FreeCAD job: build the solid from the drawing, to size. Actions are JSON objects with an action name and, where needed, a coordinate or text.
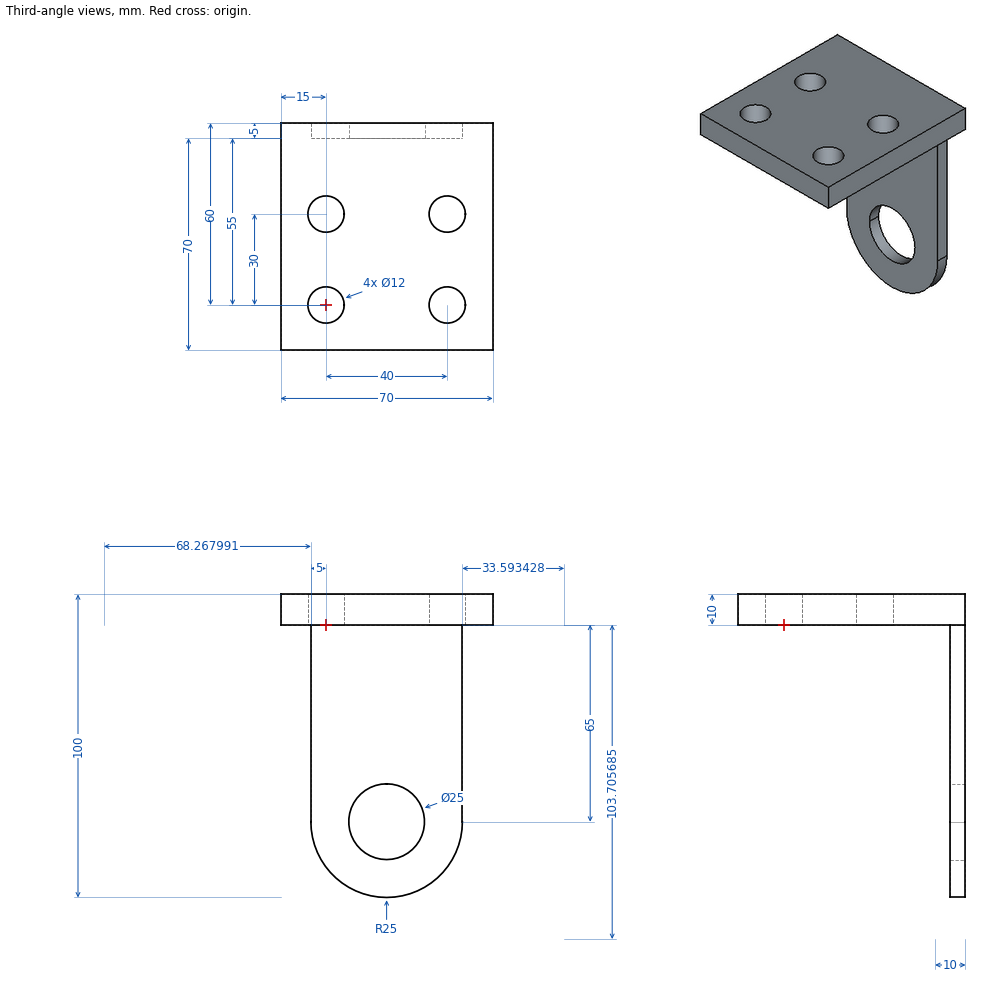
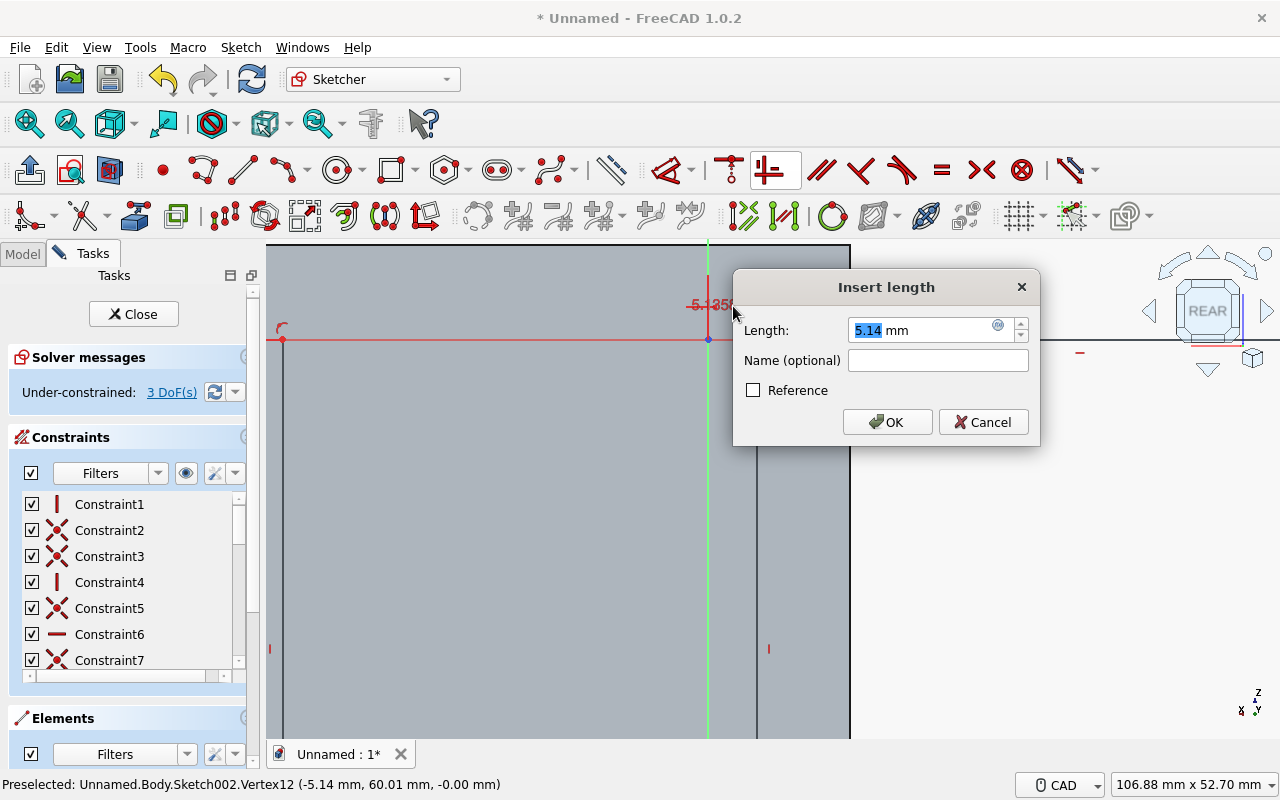
{"action": "type", "text": "5"}
{"action": "key", "text": "Return"}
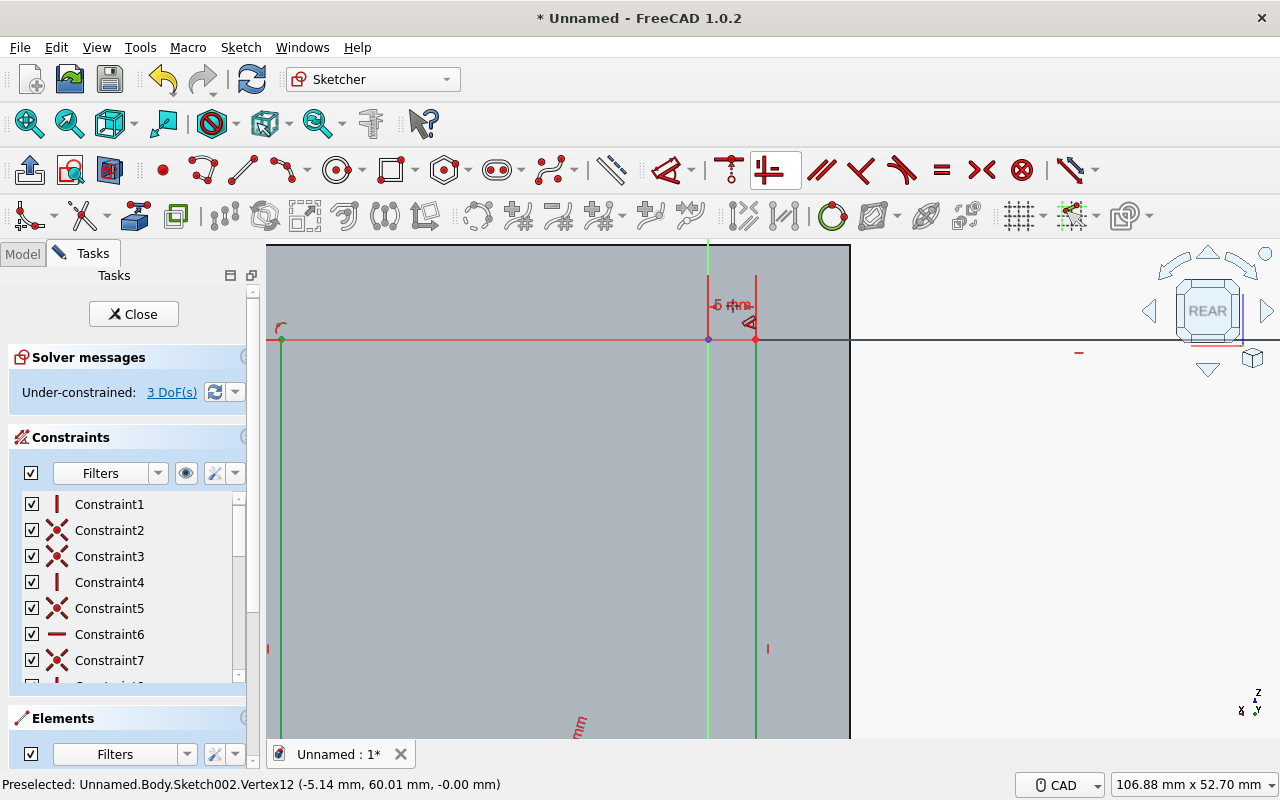
{"action": "scroll", "coordinate": [714, 341], "scroll_direction": "down", "scroll_amount": 6}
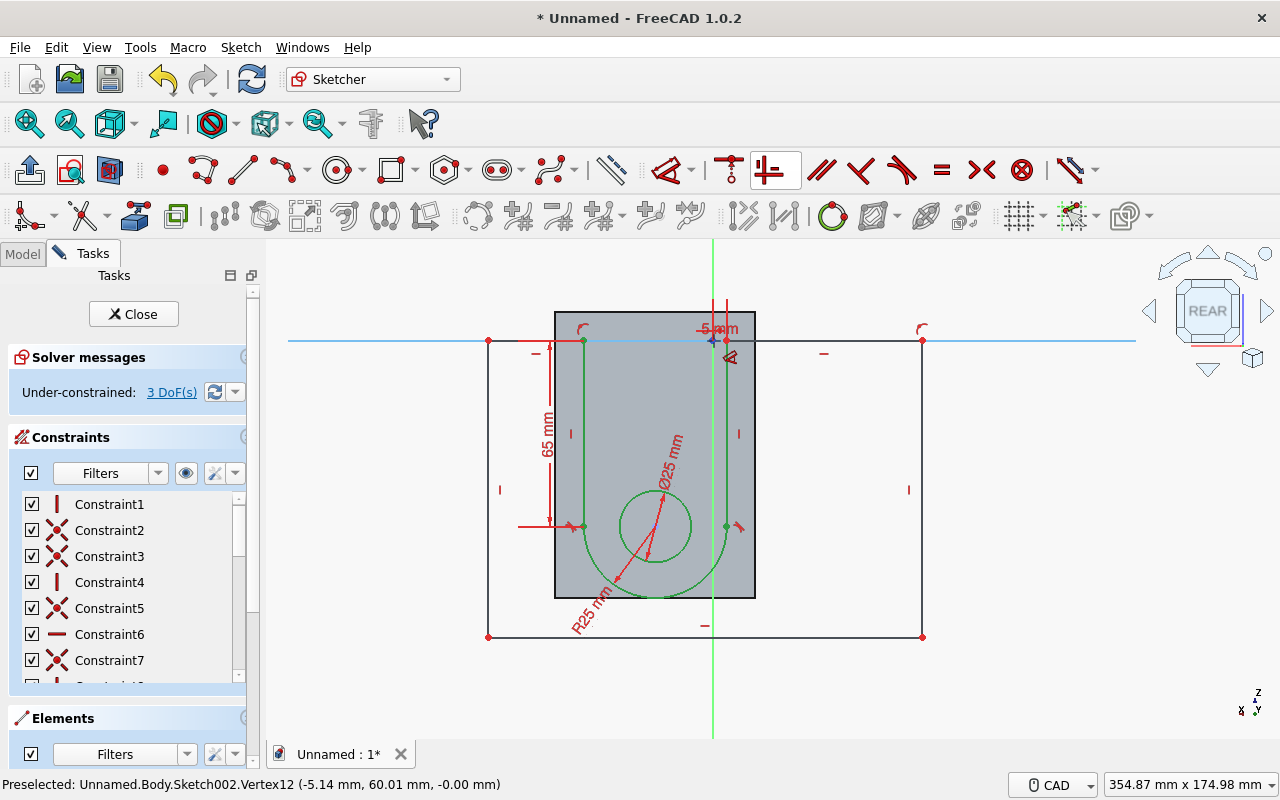
{"action": "left_click", "coordinate": [555, 341]}
{"action": "left_click", "coordinate": [536, 307]}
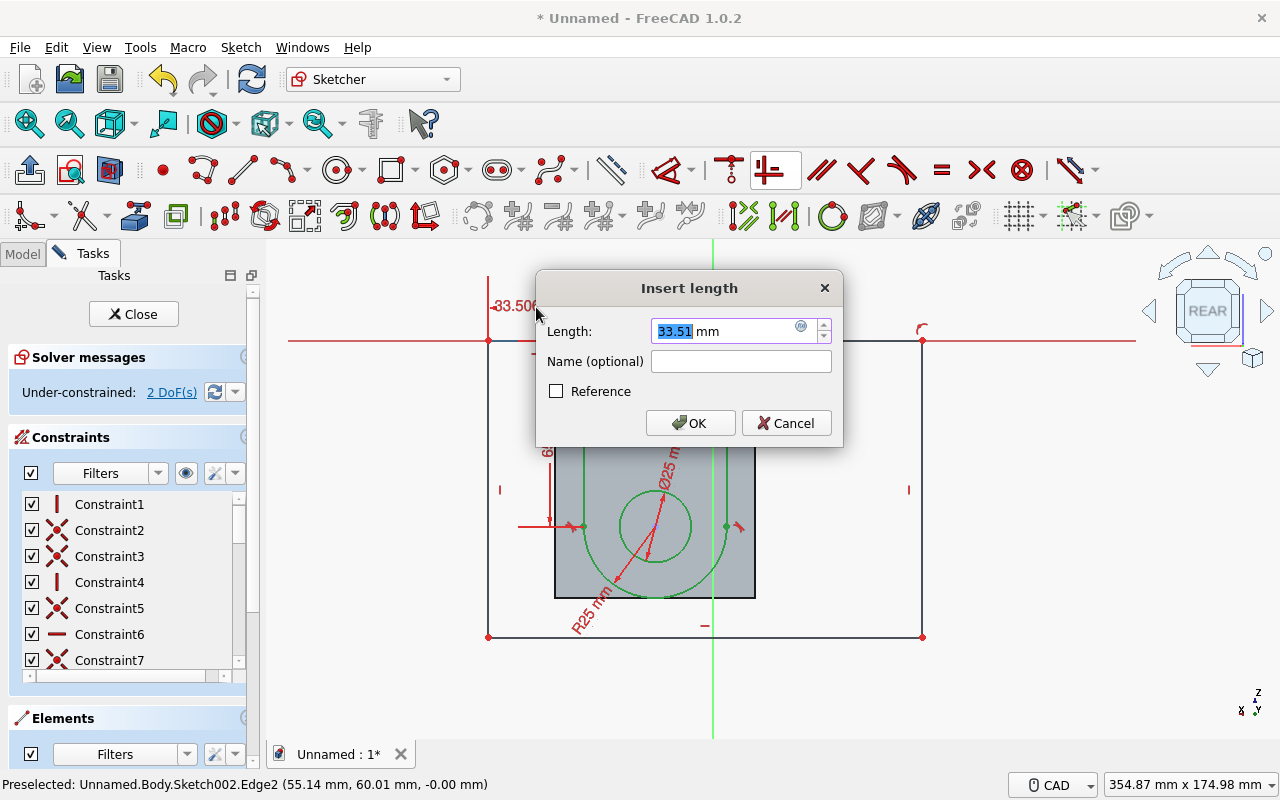
{"action": "type", "text": "33.593428"}
{"action": "key", "text": "Return"}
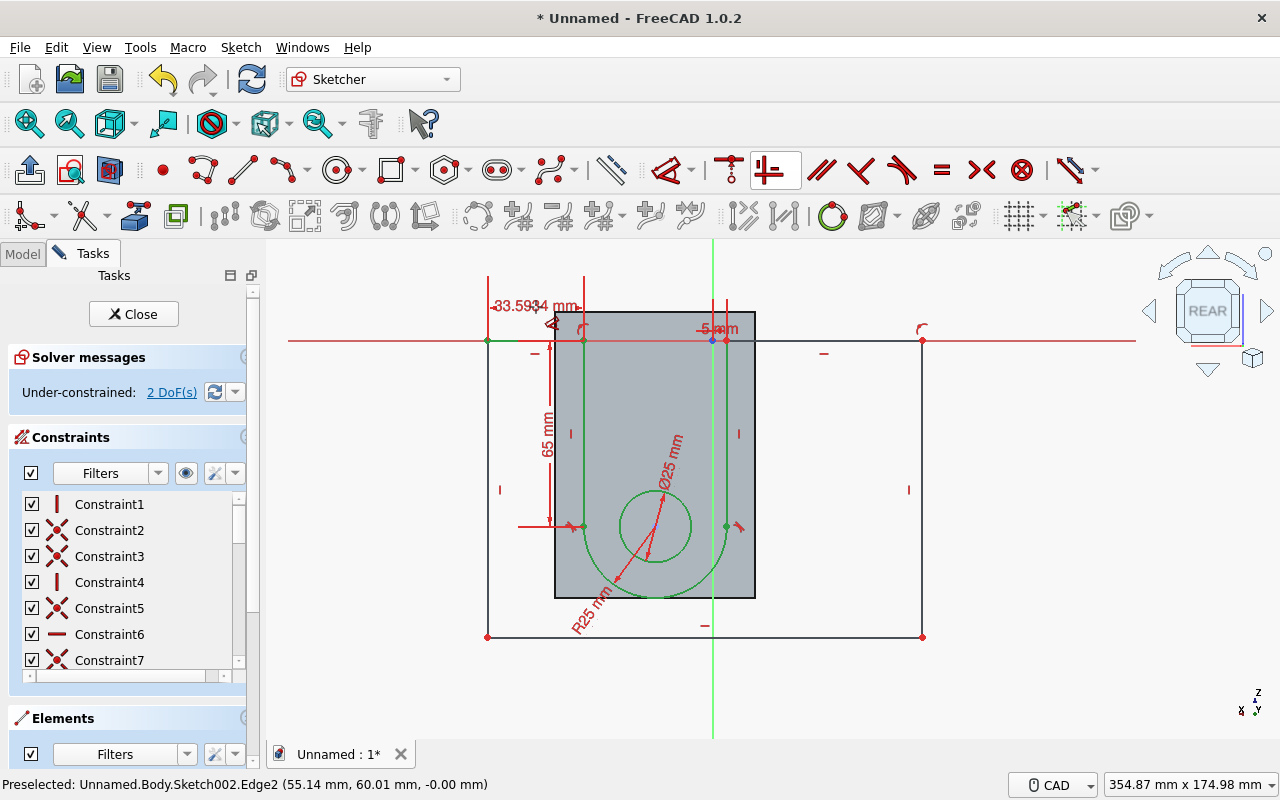
{"action": "left_click", "coordinate": [864, 341]}
{"action": "left_click", "coordinate": [825, 307]}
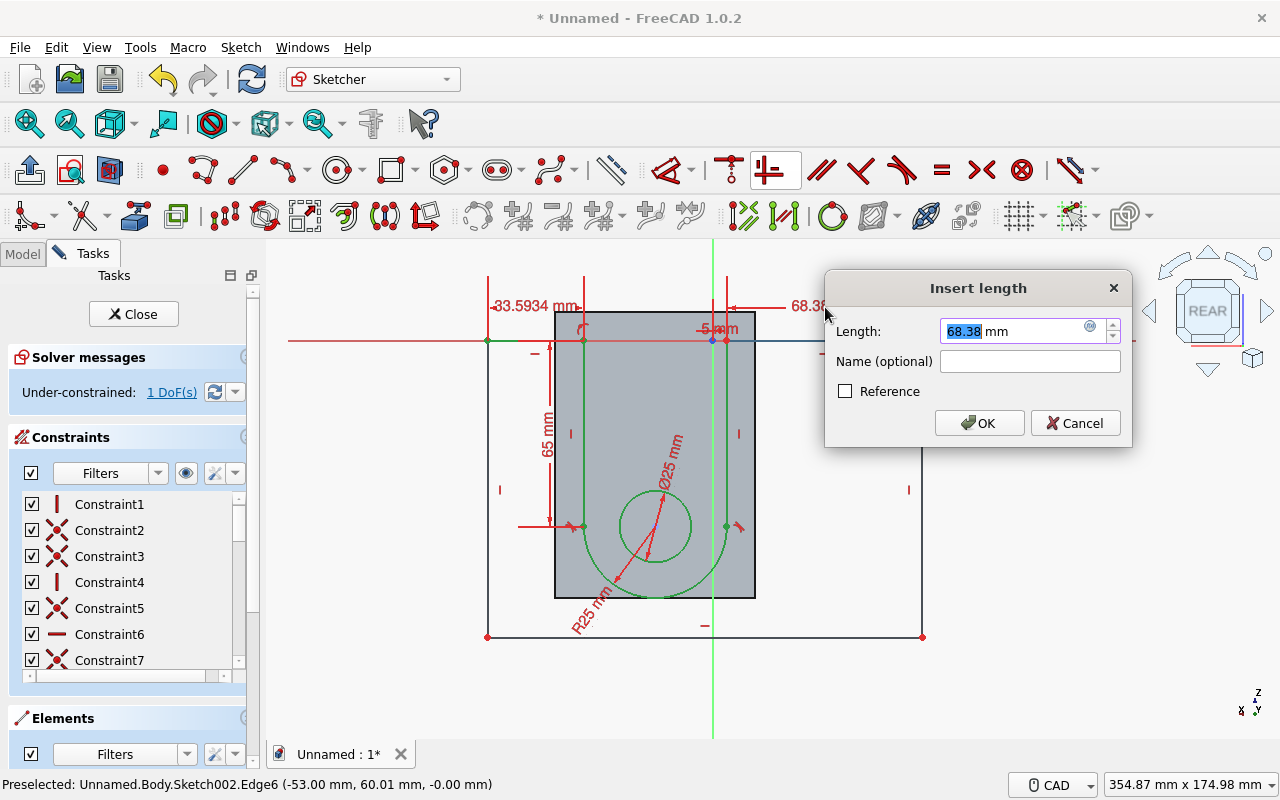
{"action": "type", "text": "68.267991"}
{"action": "key", "text": "Return"}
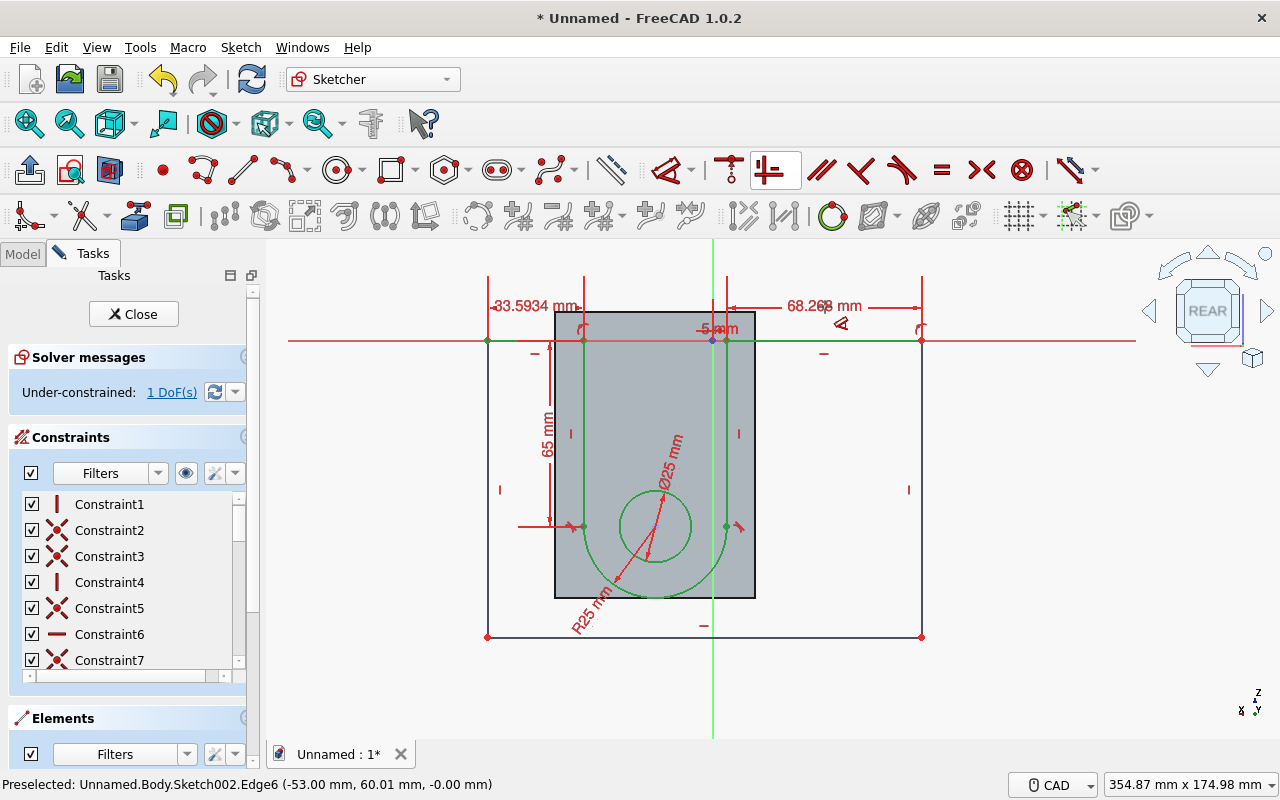
{"action": "left_click", "coordinate": [488, 430]}
{"action": "left_click", "coordinate": [454, 489]}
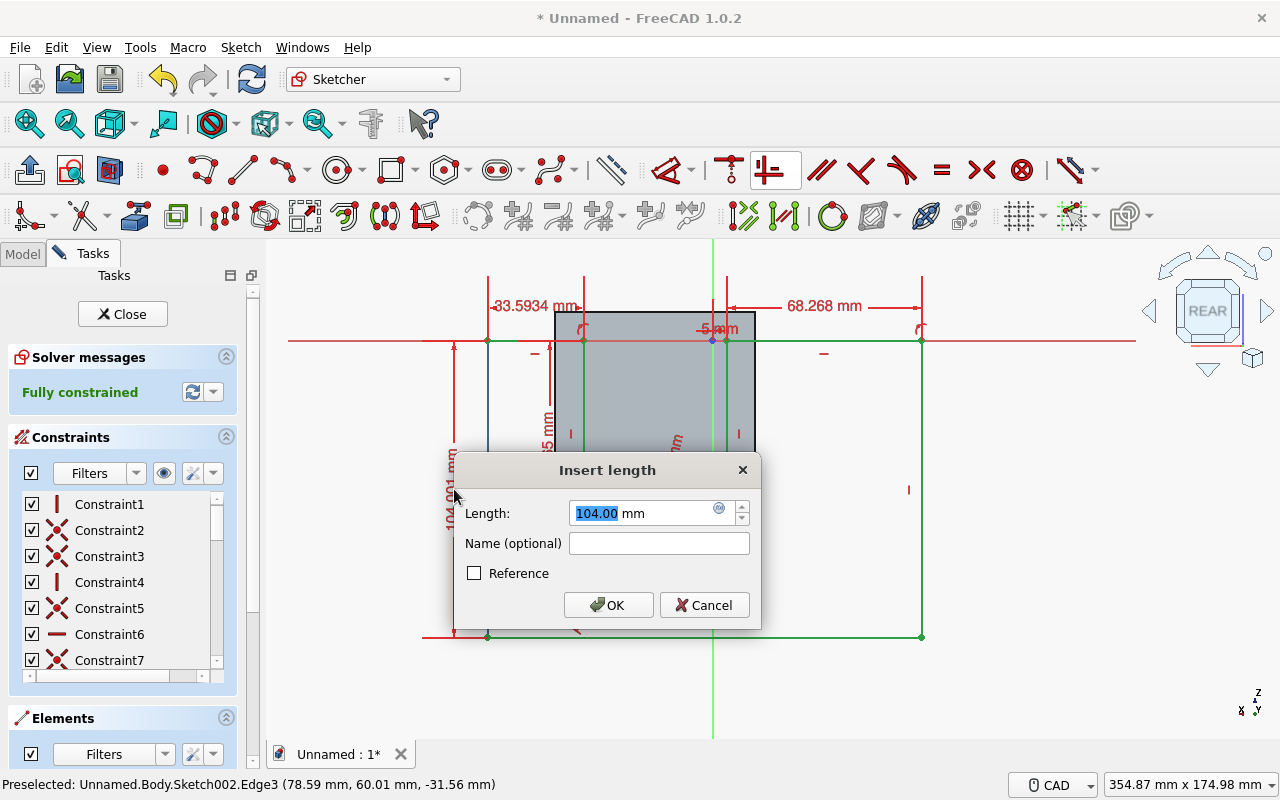
{"action": "type", "text": "103.705685"}
{"action": "key", "text": "Return"}
{"action": "key", "text": "Escape"}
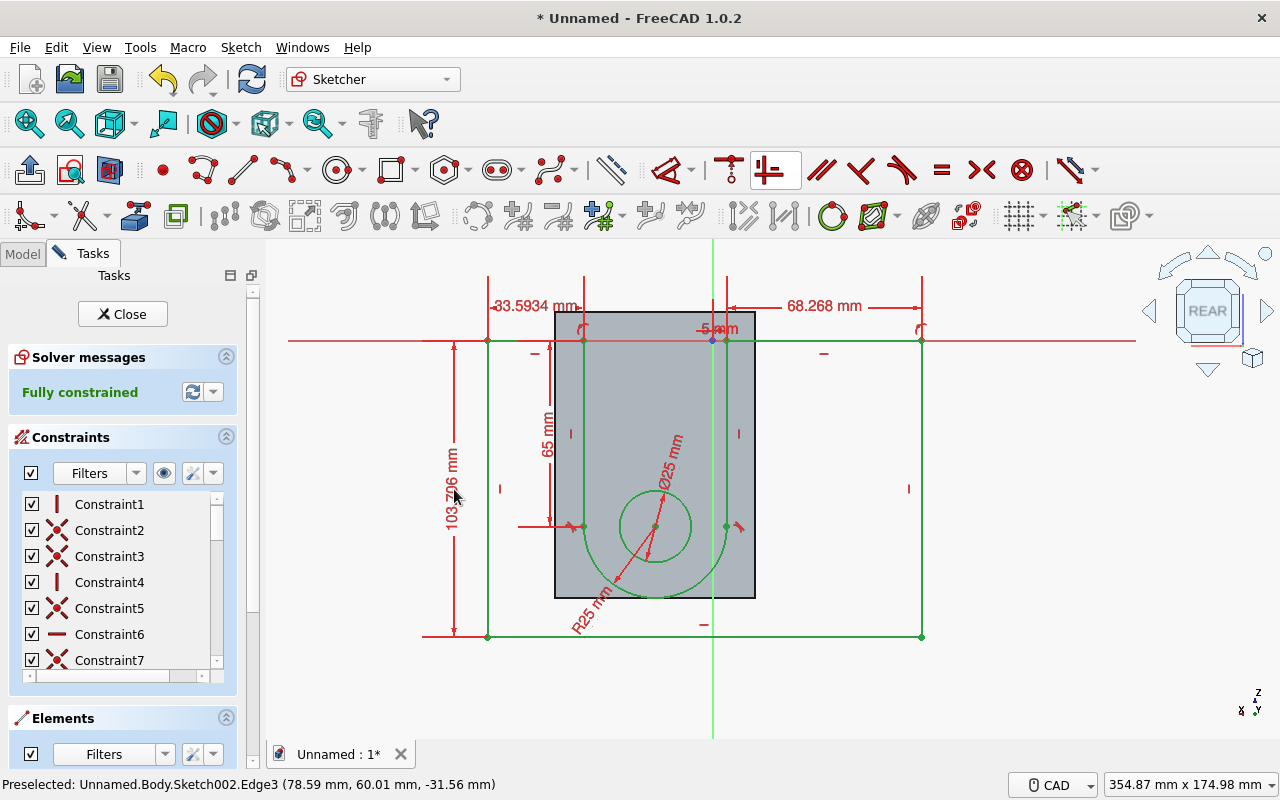
{"action": "left_click", "coordinate": [123, 314]}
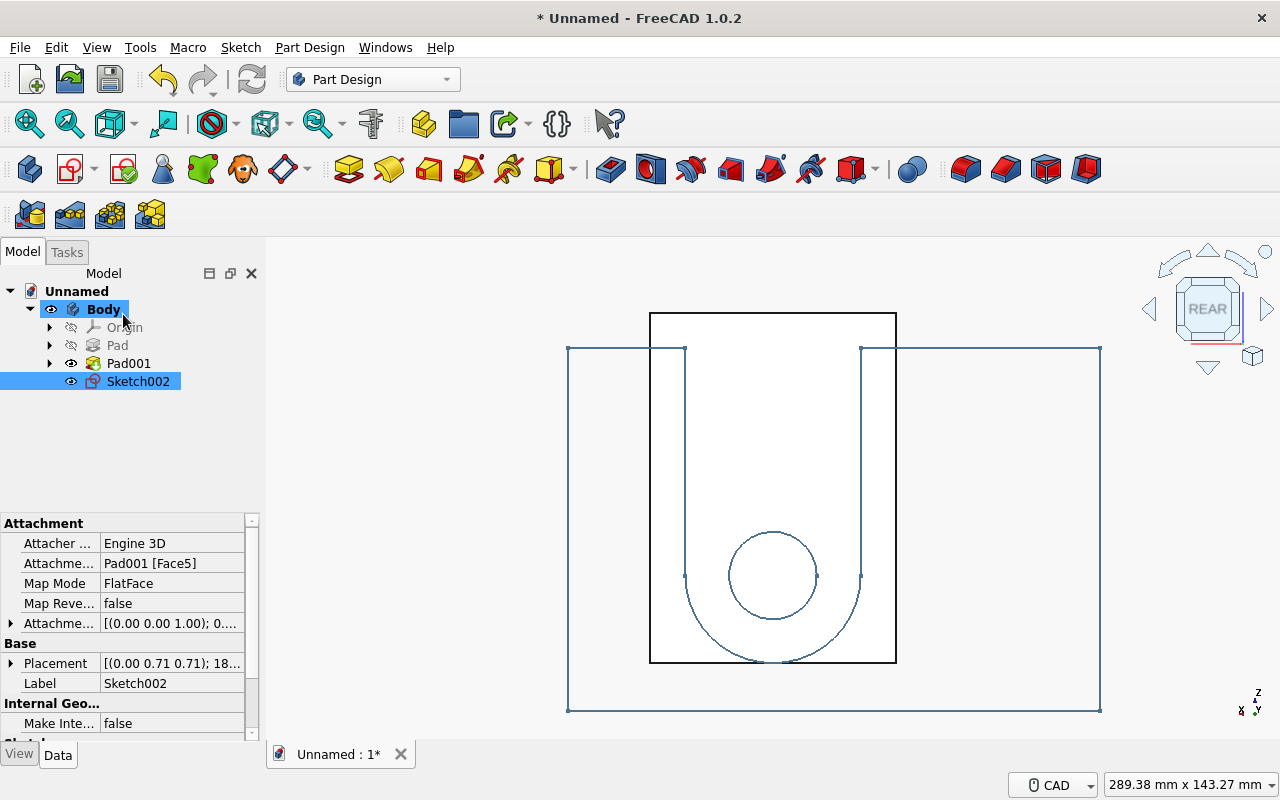
{"action": "left_click", "coordinate": [612, 170]}